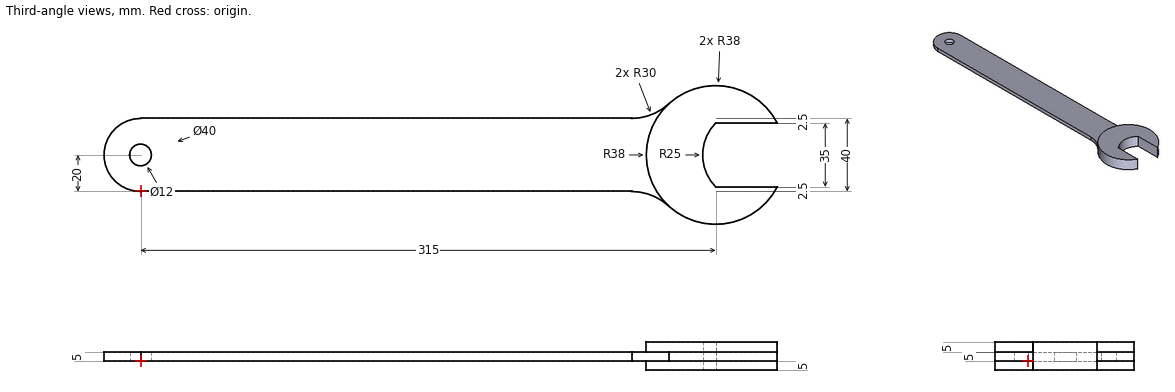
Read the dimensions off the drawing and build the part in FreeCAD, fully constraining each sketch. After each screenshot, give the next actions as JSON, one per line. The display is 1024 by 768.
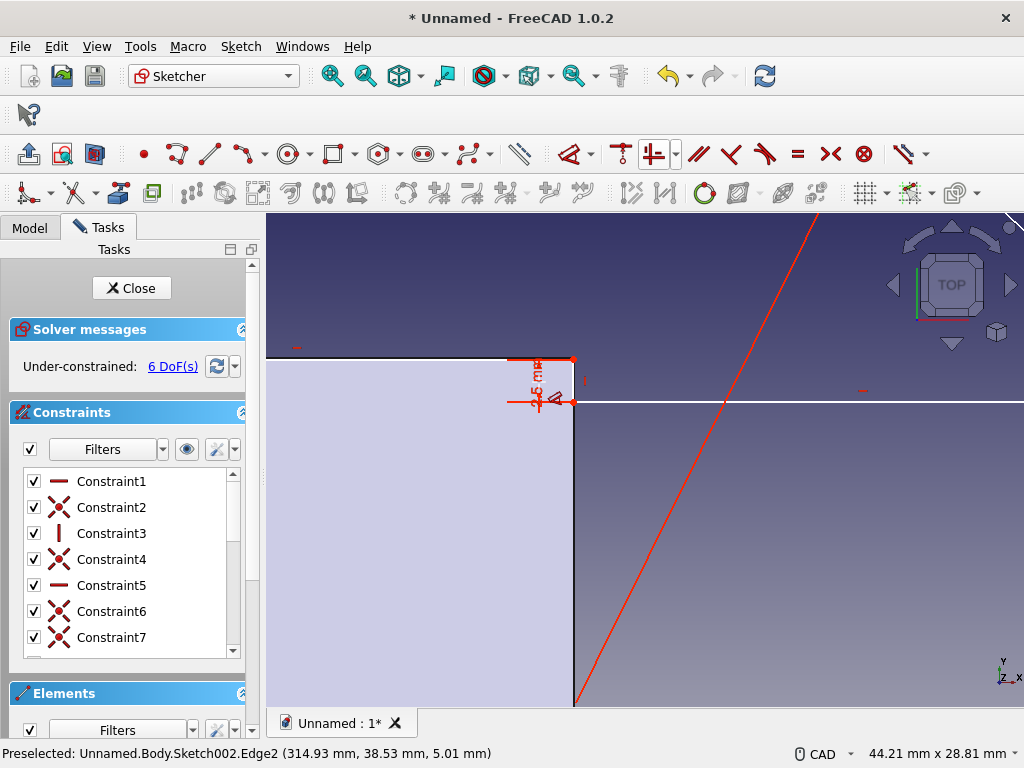
{"action": "scroll", "coordinate": [573, 381], "scroll_direction": "down", "scroll_amount": 7}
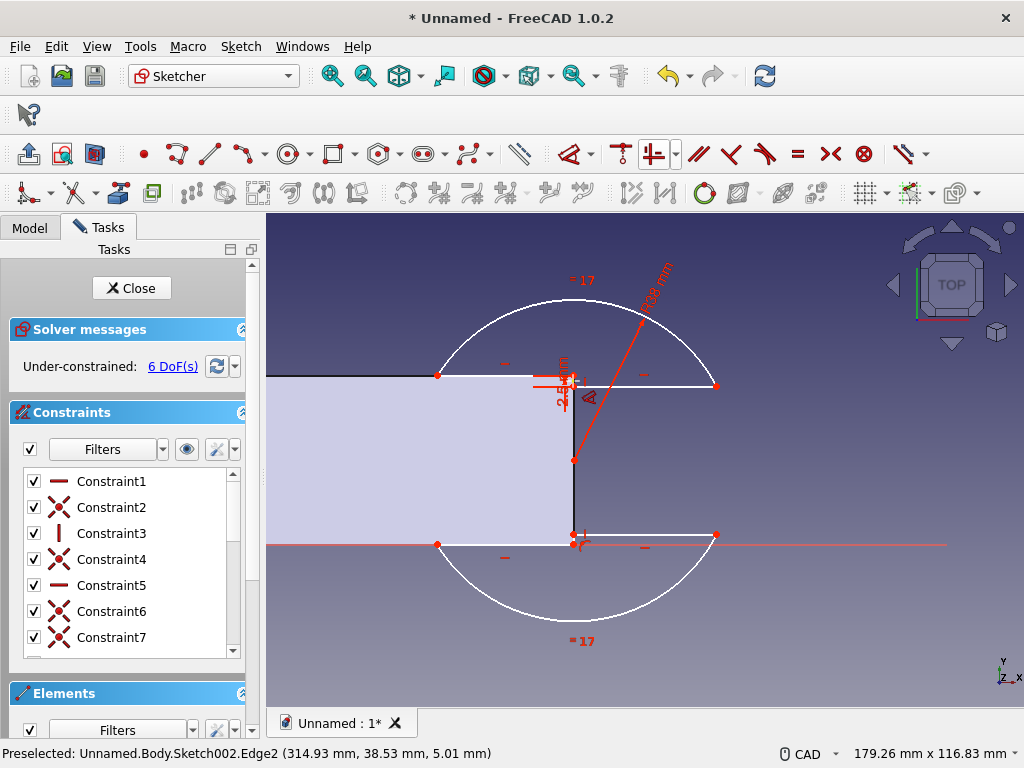
{"action": "scroll", "coordinate": [574, 538], "scroll_direction": "up", "scroll_amount": 8}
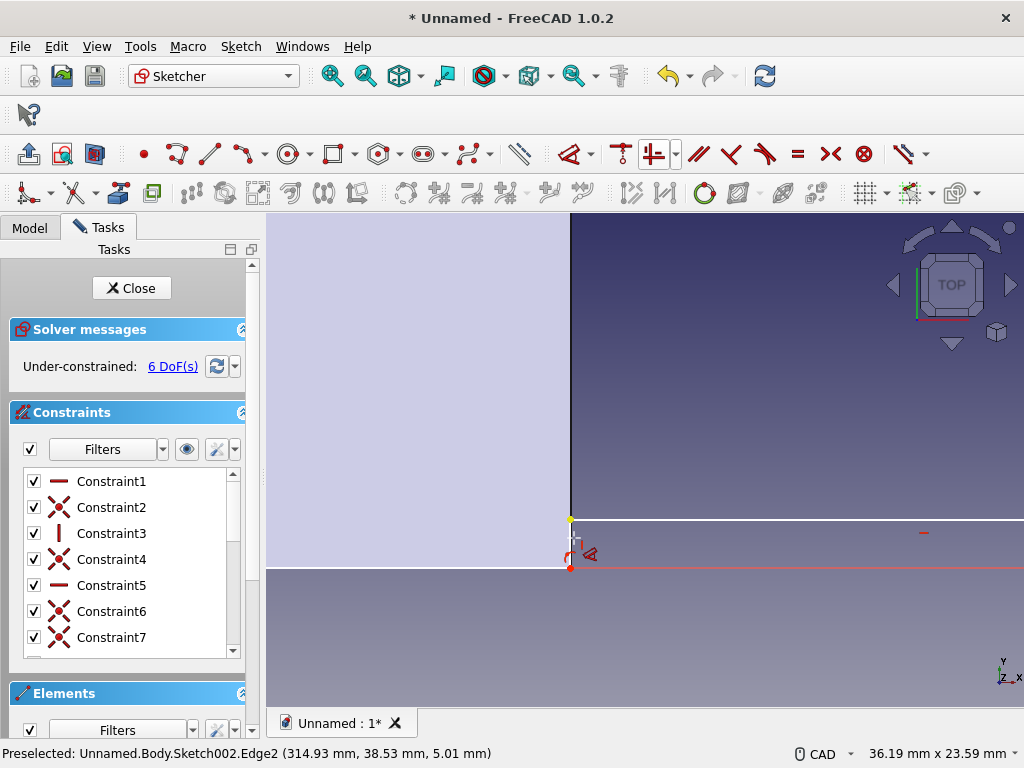
{"action": "left_click", "coordinate": [570, 534]}
{"action": "left_click", "coordinate": [536, 544]}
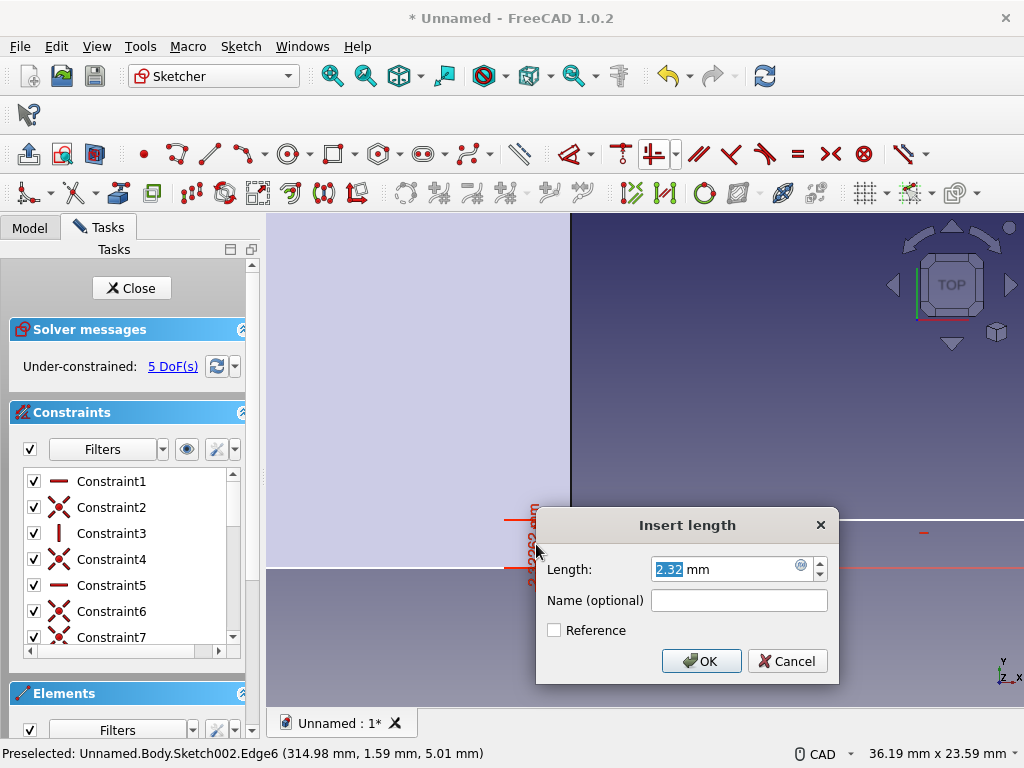
{"action": "type", "text": "2.5"}
{"action": "key", "text": "Return"}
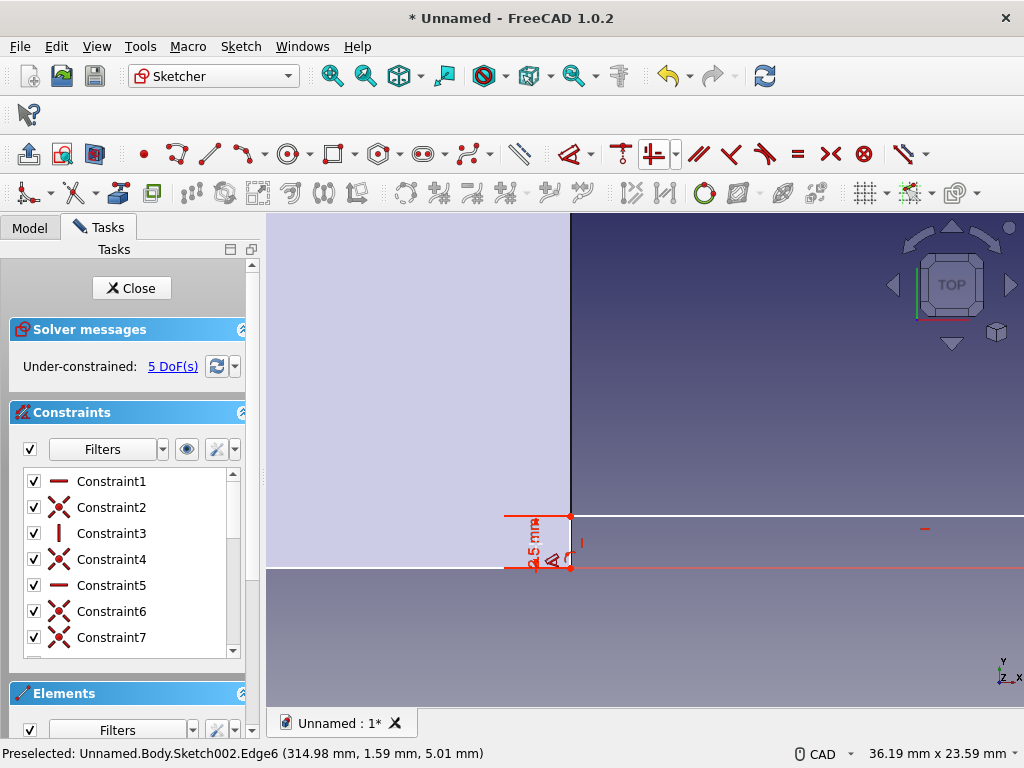
{"action": "scroll", "coordinate": [574, 539], "scroll_direction": "down", "scroll_amount": 8}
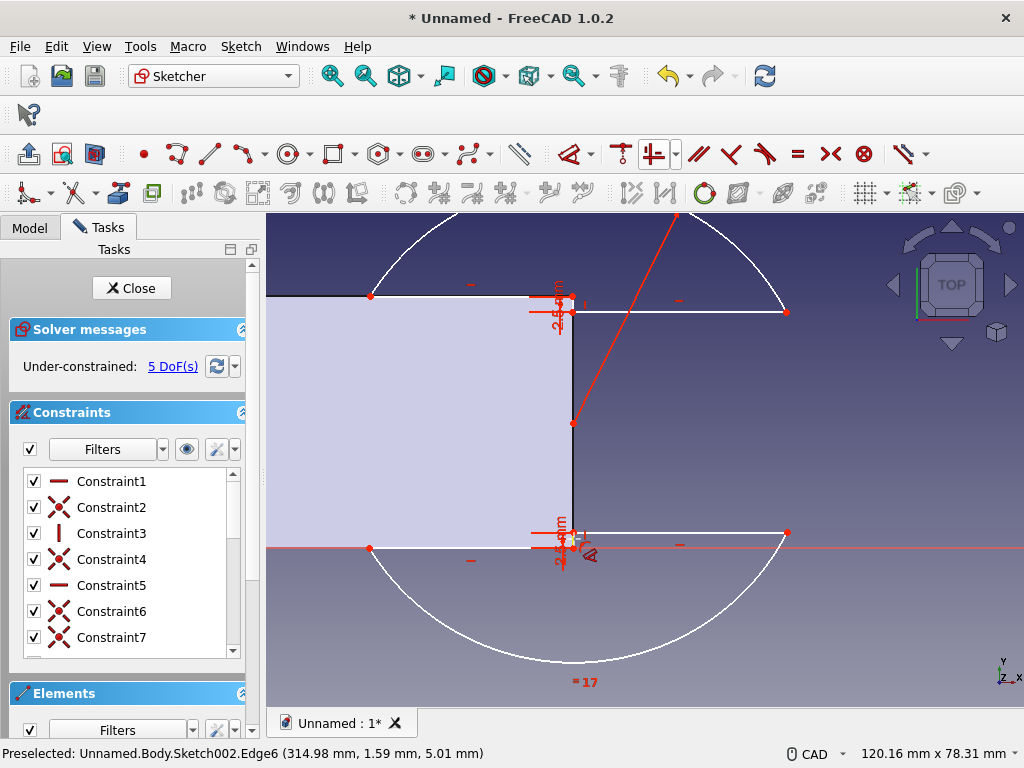
{"action": "left_click", "coordinate": [437, 377]}
{"action": "left_click", "coordinate": [471, 461]}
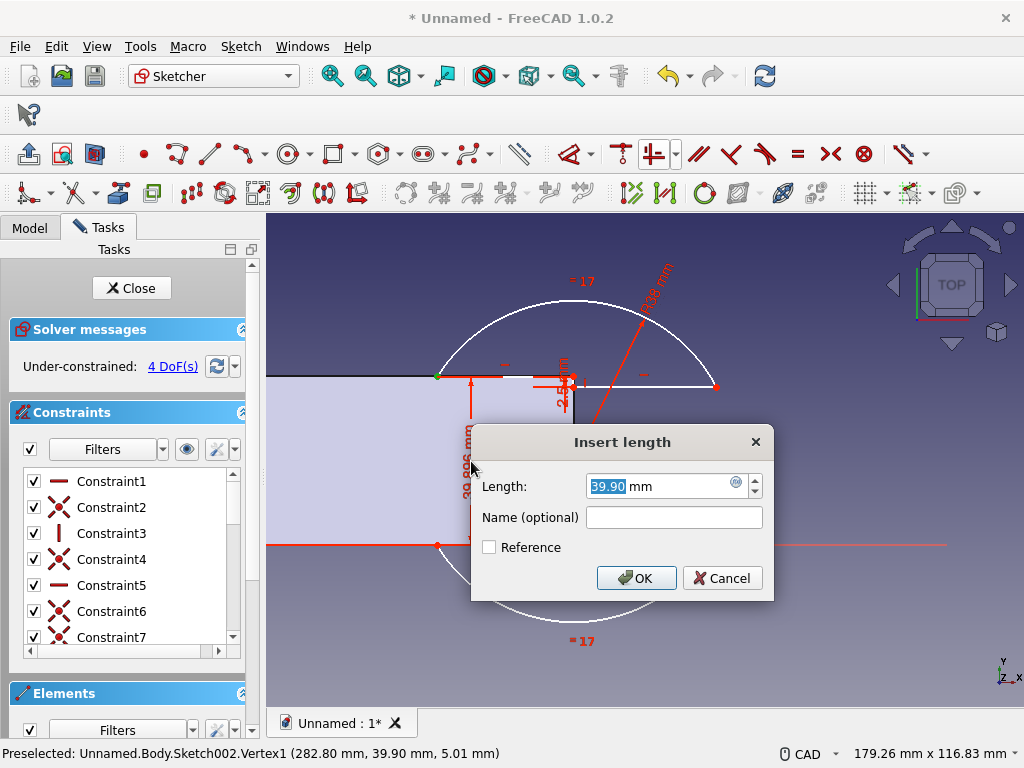
{"action": "type", "text": "40"}
{"action": "key", "text": "Return"}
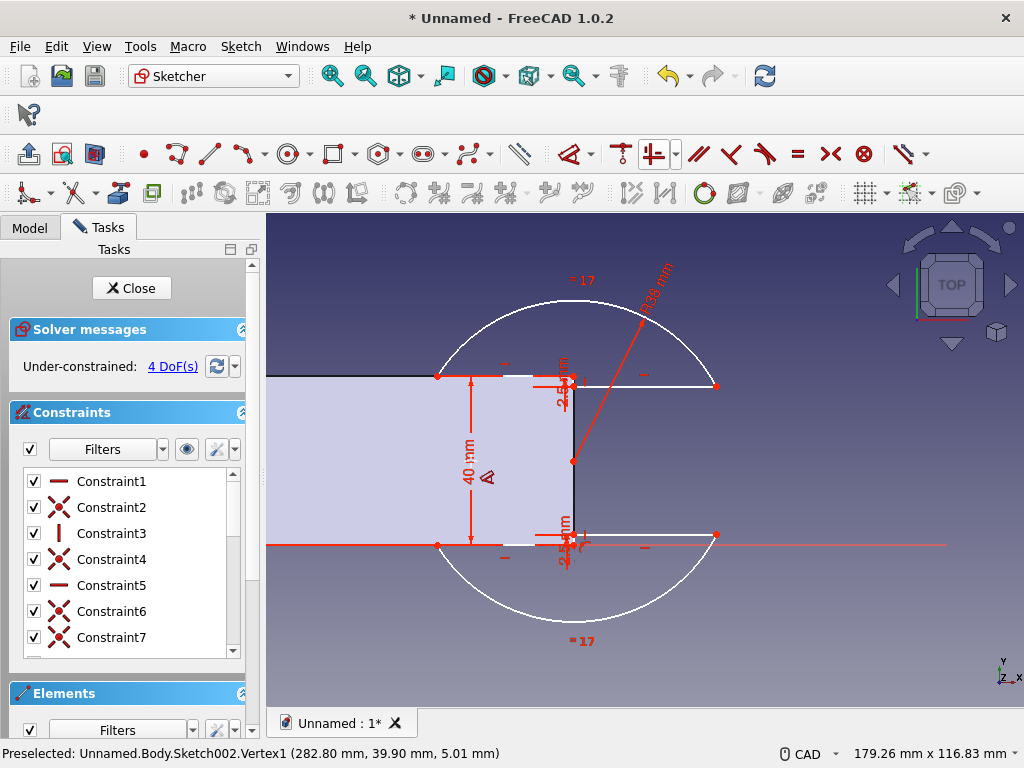
{"action": "left_click", "coordinate": [574, 461]}
{"action": "left_click", "coordinate": [608, 503]}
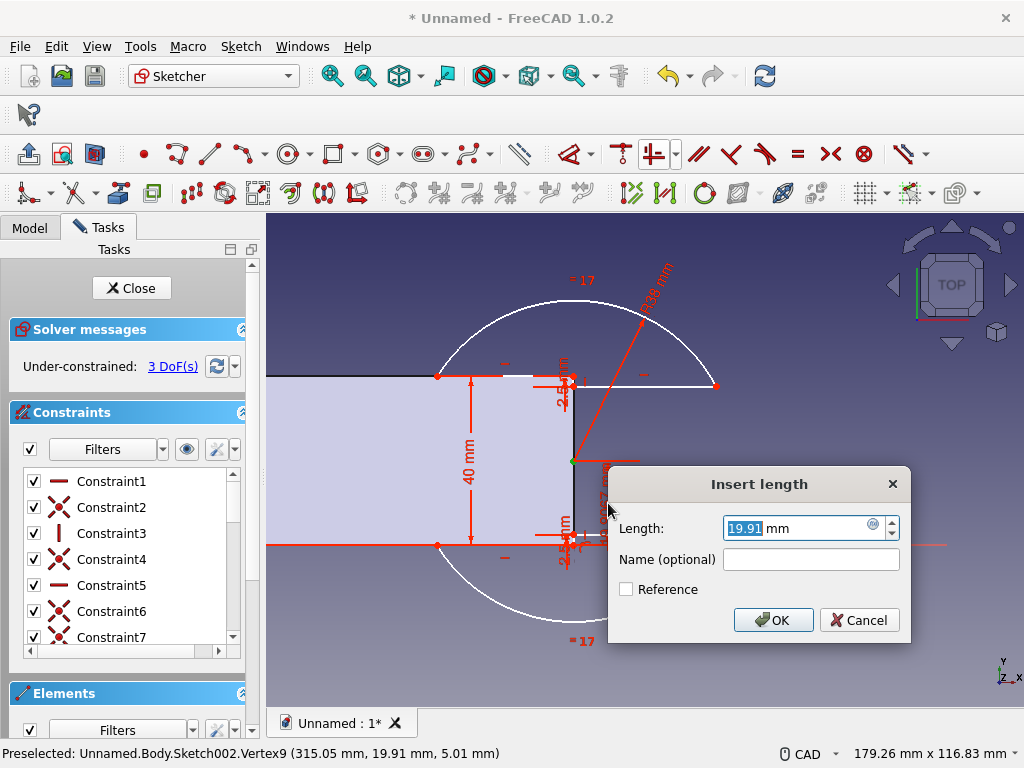
{"action": "type", "text": "20"}
{"action": "key", "text": "Return"}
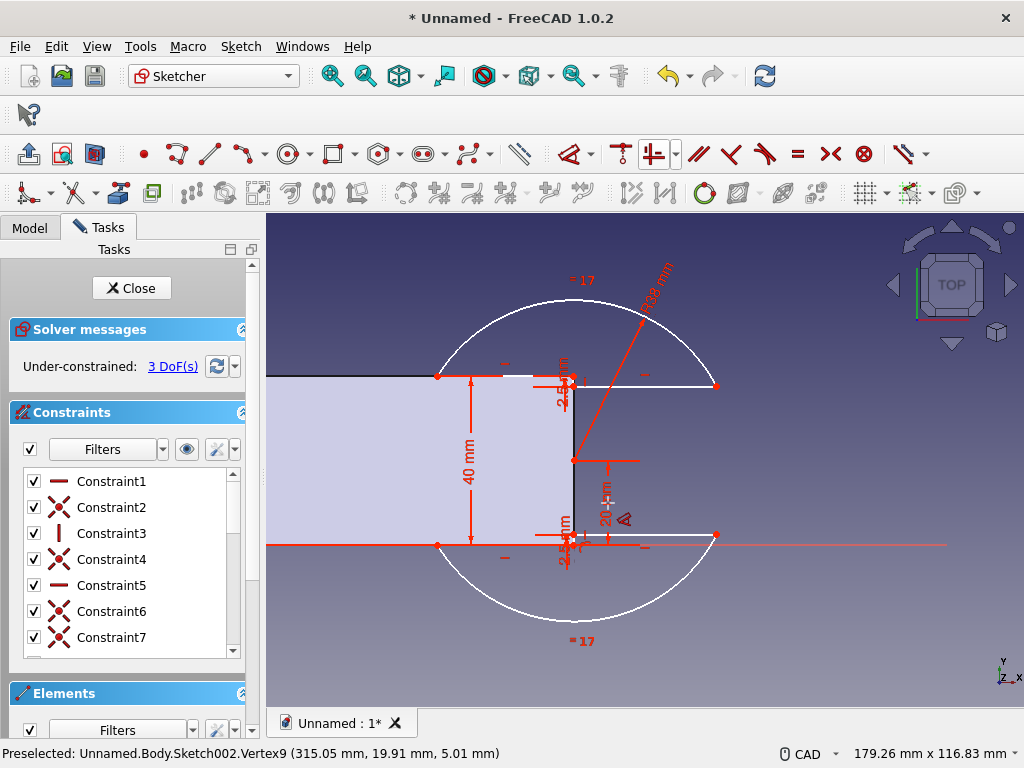
{"action": "left_click", "coordinate": [573, 376]}
{"action": "left_click", "coordinate": [434, 579]}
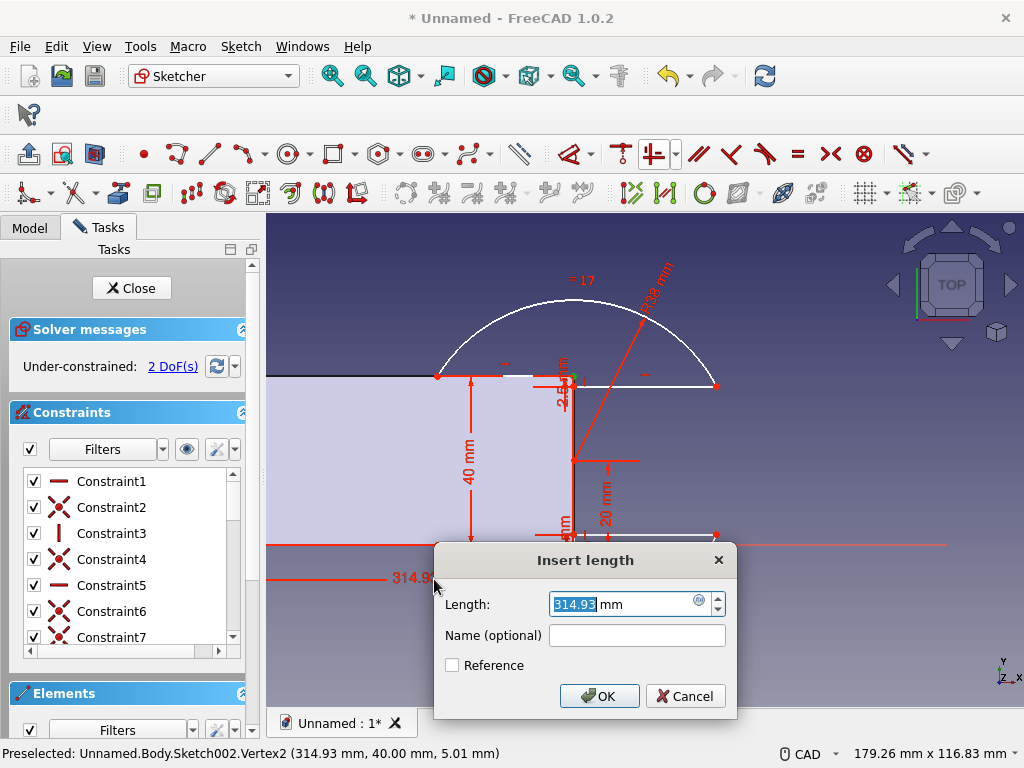
{"action": "type", "text": "315"}
{"action": "key", "text": "Return"}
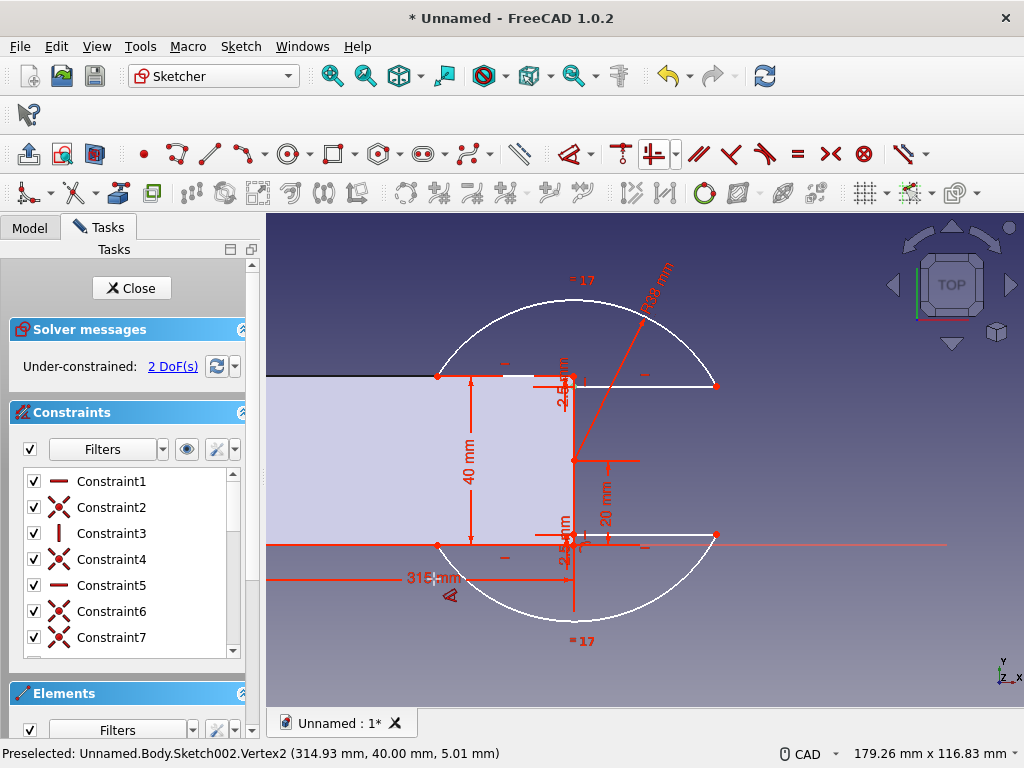
{"action": "left_click", "coordinate": [574, 535]}
{"action": "left_click", "coordinate": [336, 579]}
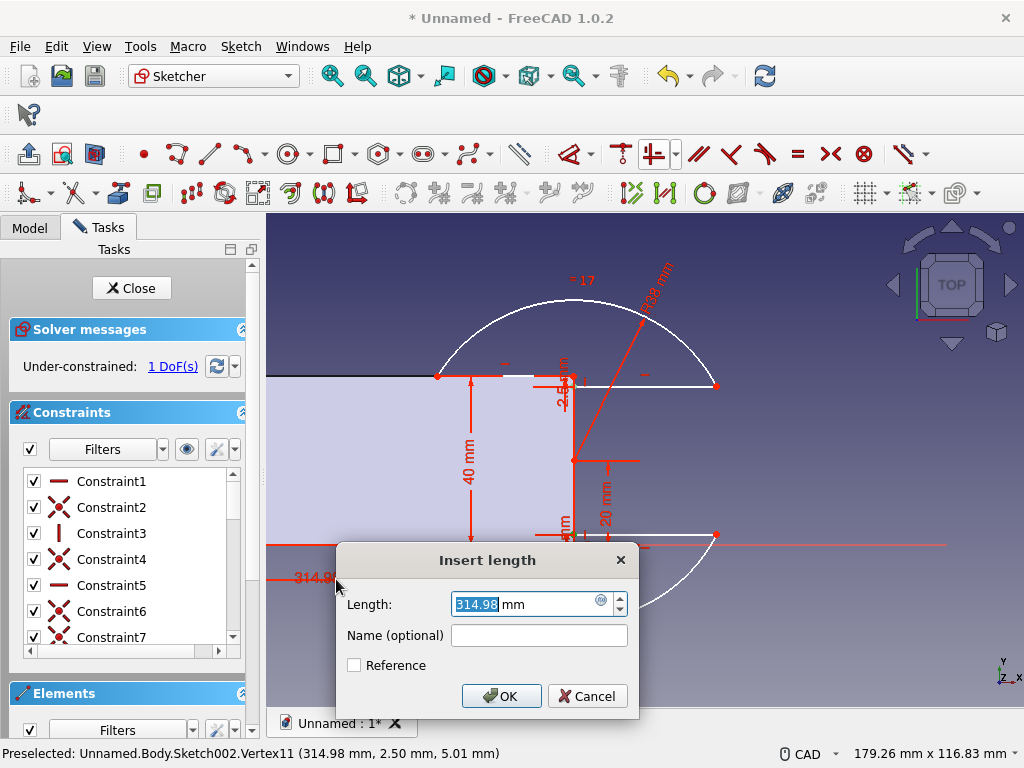
{"action": "type", "text": "315"}
{"action": "key", "text": "Return"}